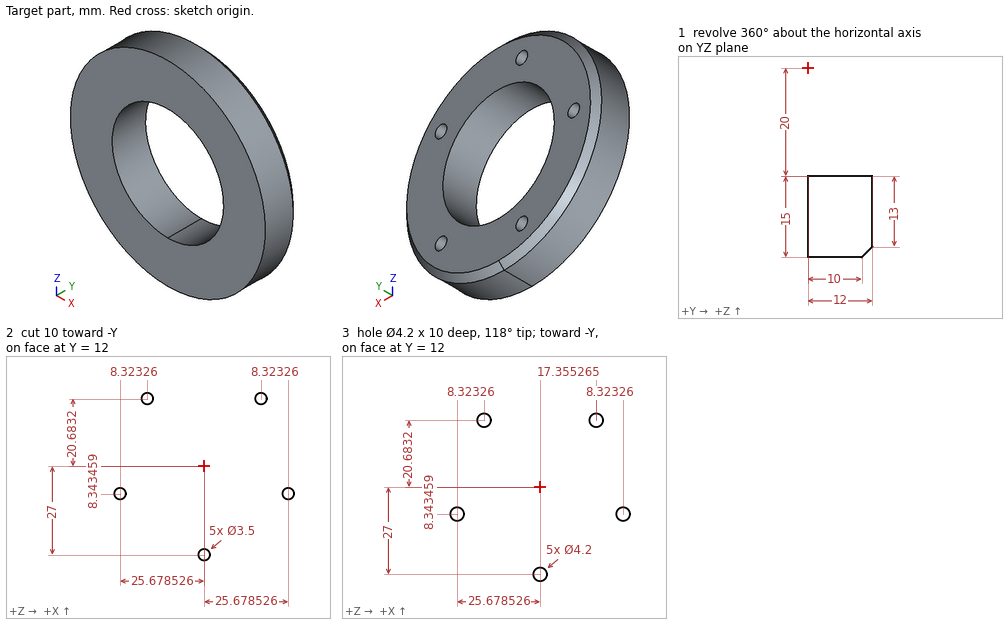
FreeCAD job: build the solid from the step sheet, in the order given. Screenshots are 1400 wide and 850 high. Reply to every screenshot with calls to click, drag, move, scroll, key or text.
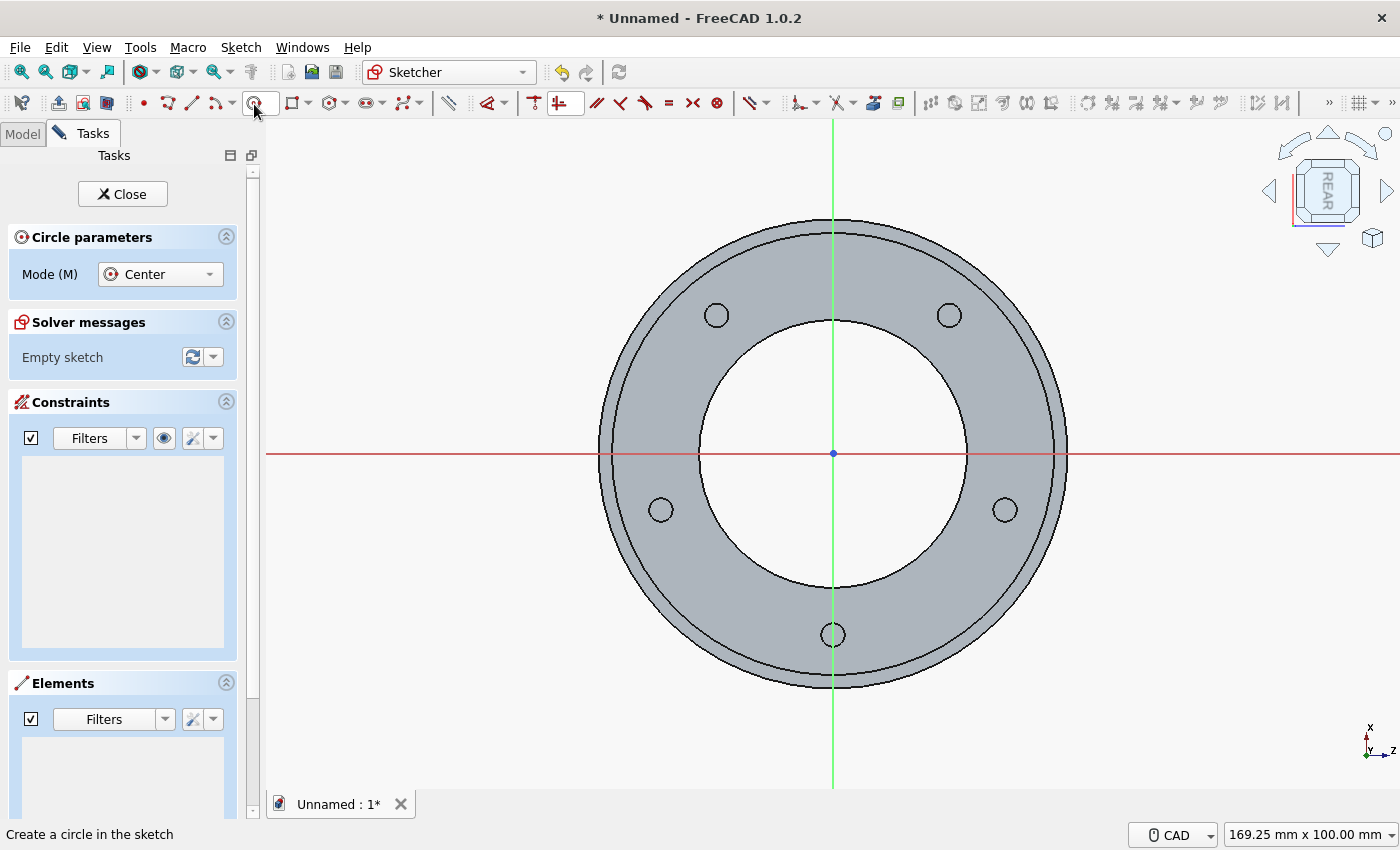
scroll(833, 635, up, 3)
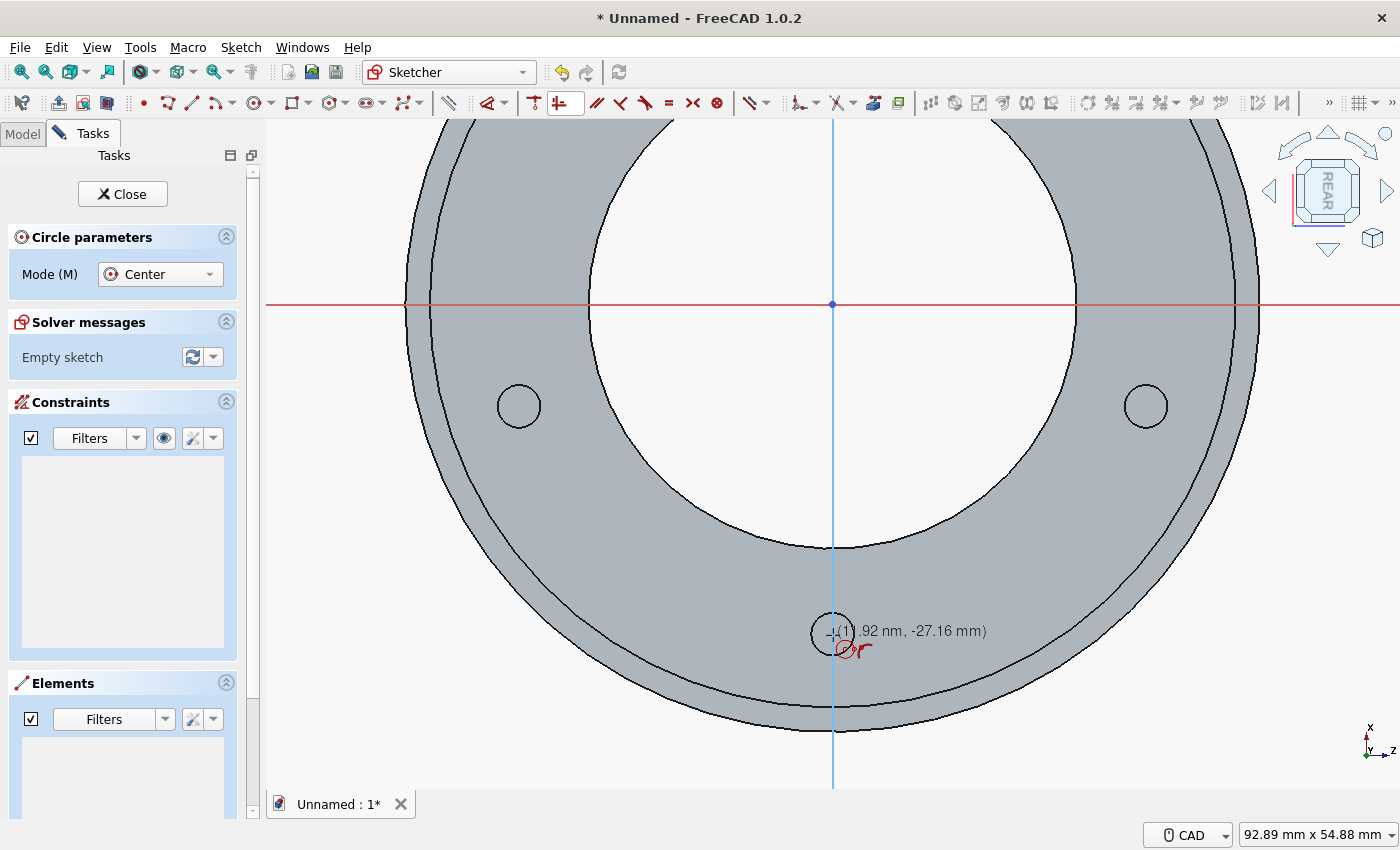
click(833, 634)
click(851, 616)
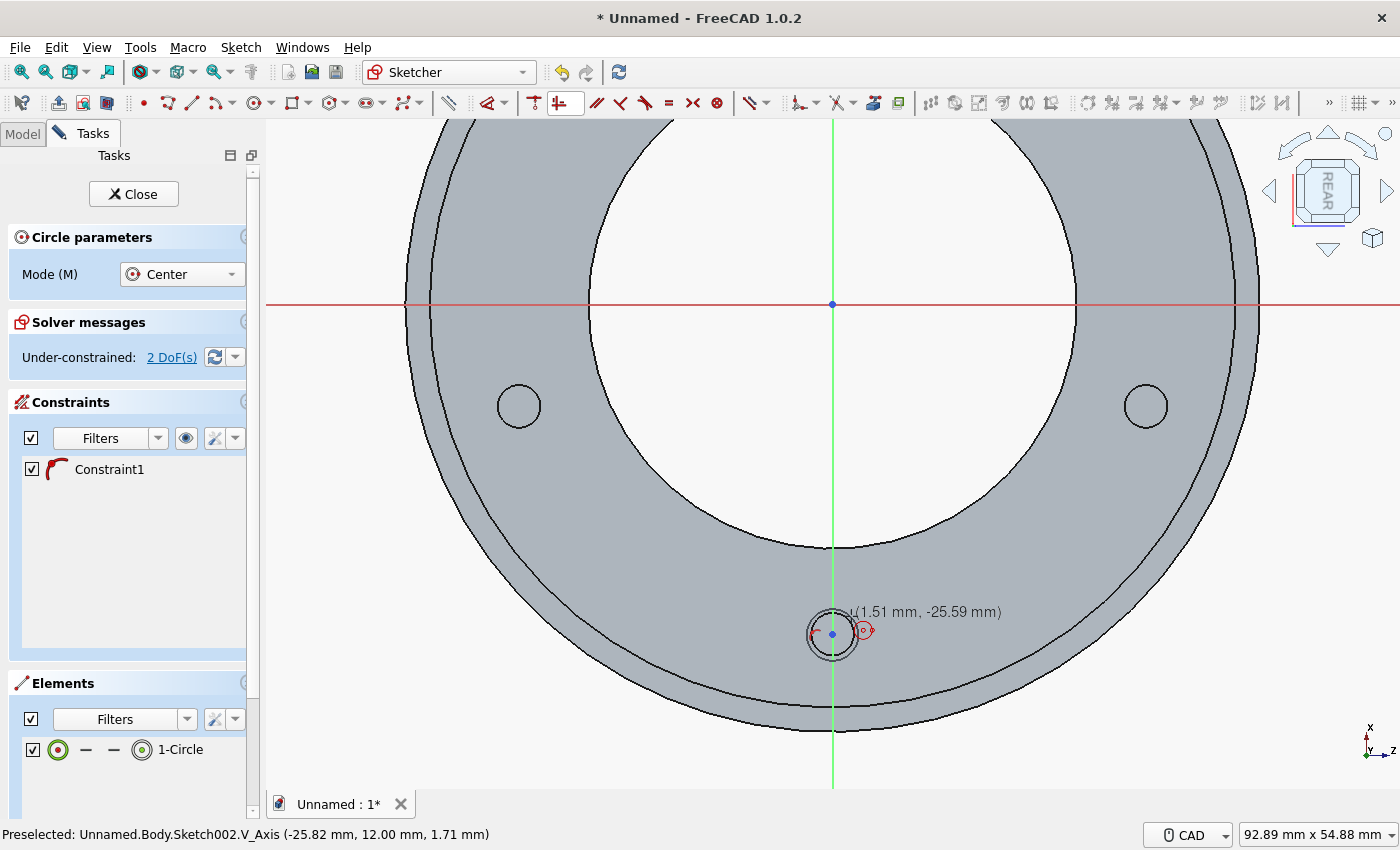
click(519, 406)
click(537, 388)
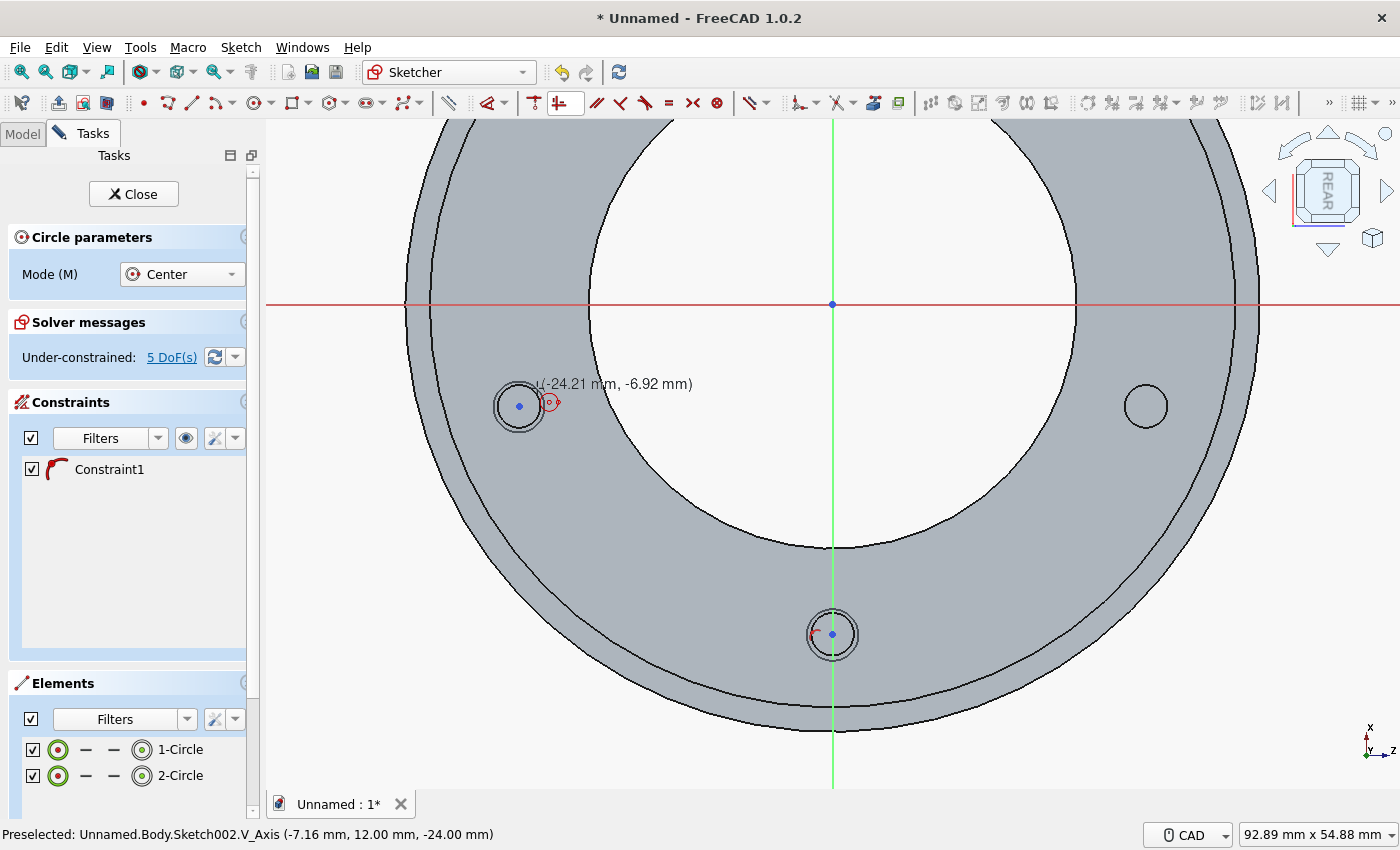
scroll(626, 679, down, 2)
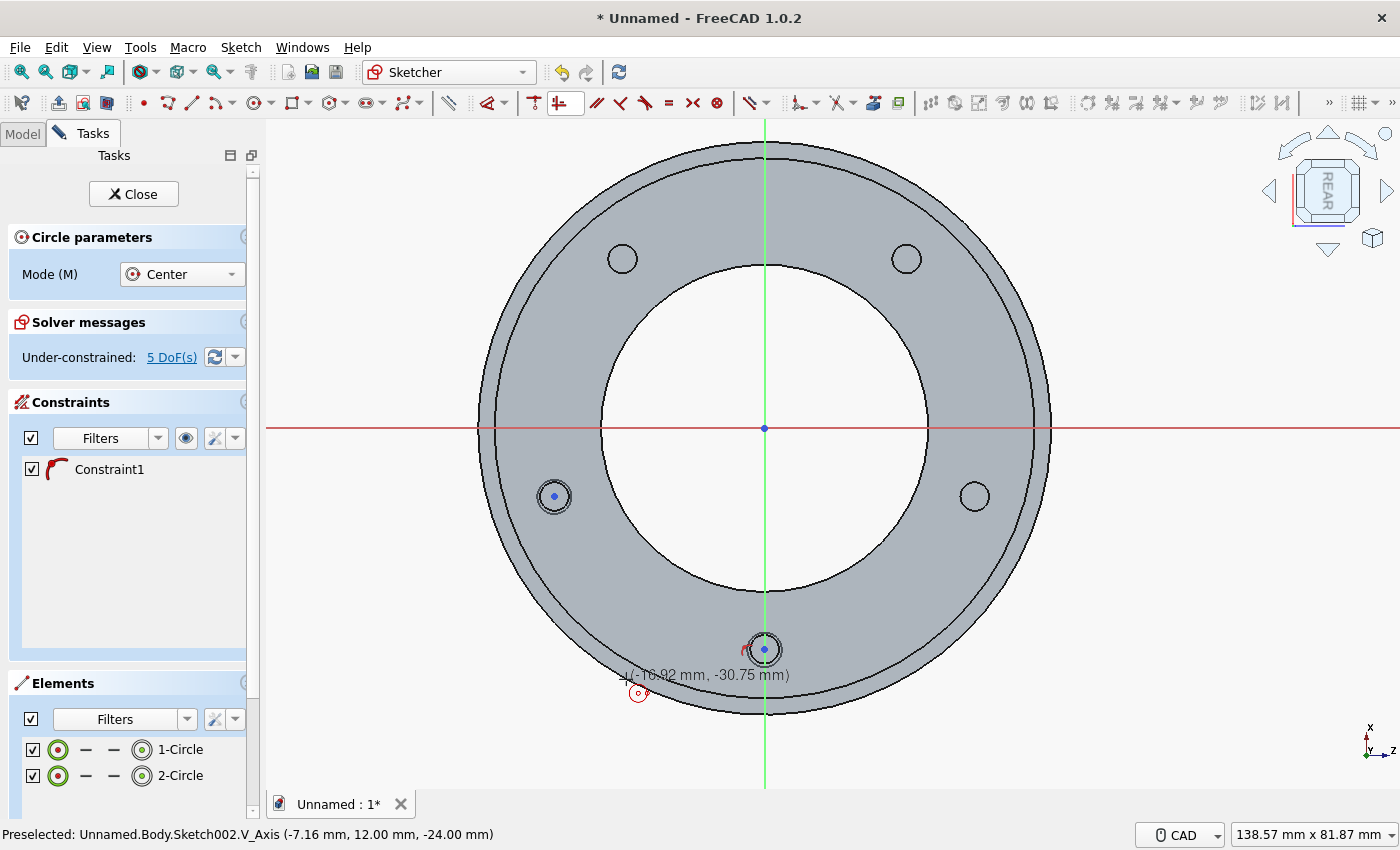
scroll(623, 259, up, 2)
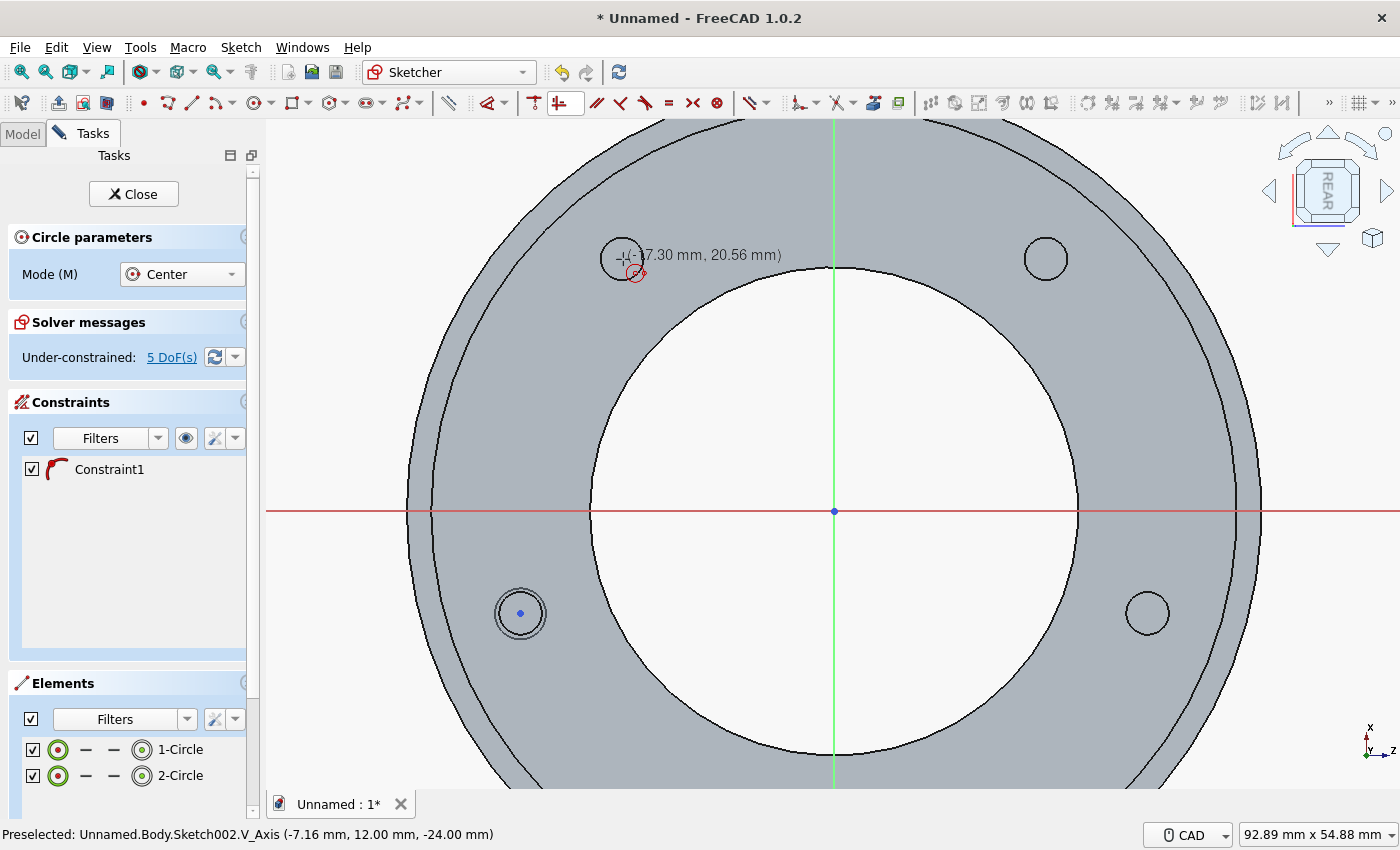
click(622, 259)
click(640, 241)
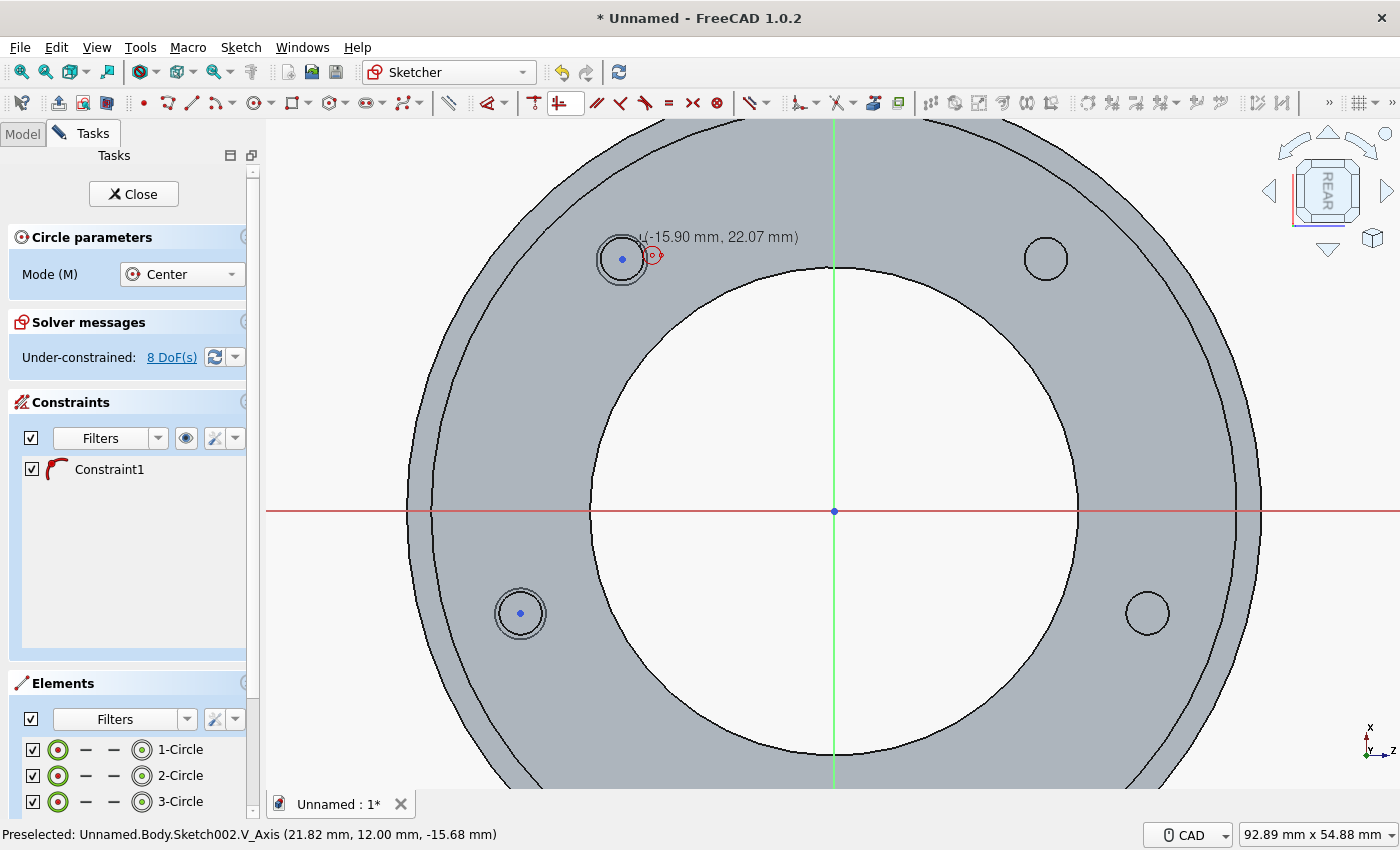
click(1046, 259)
click(1064, 241)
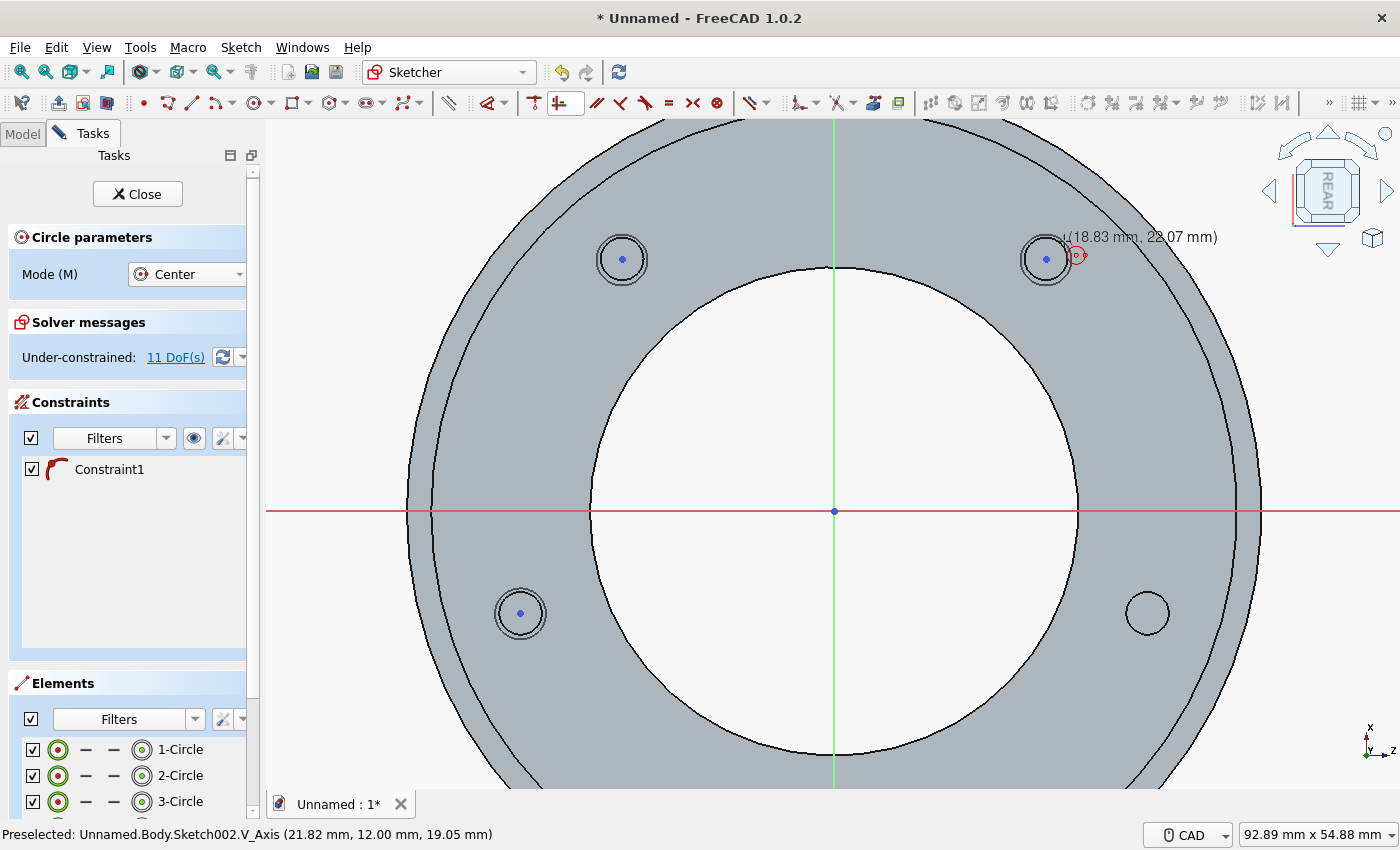
click(1148, 613)
click(1166, 595)
key(Escape)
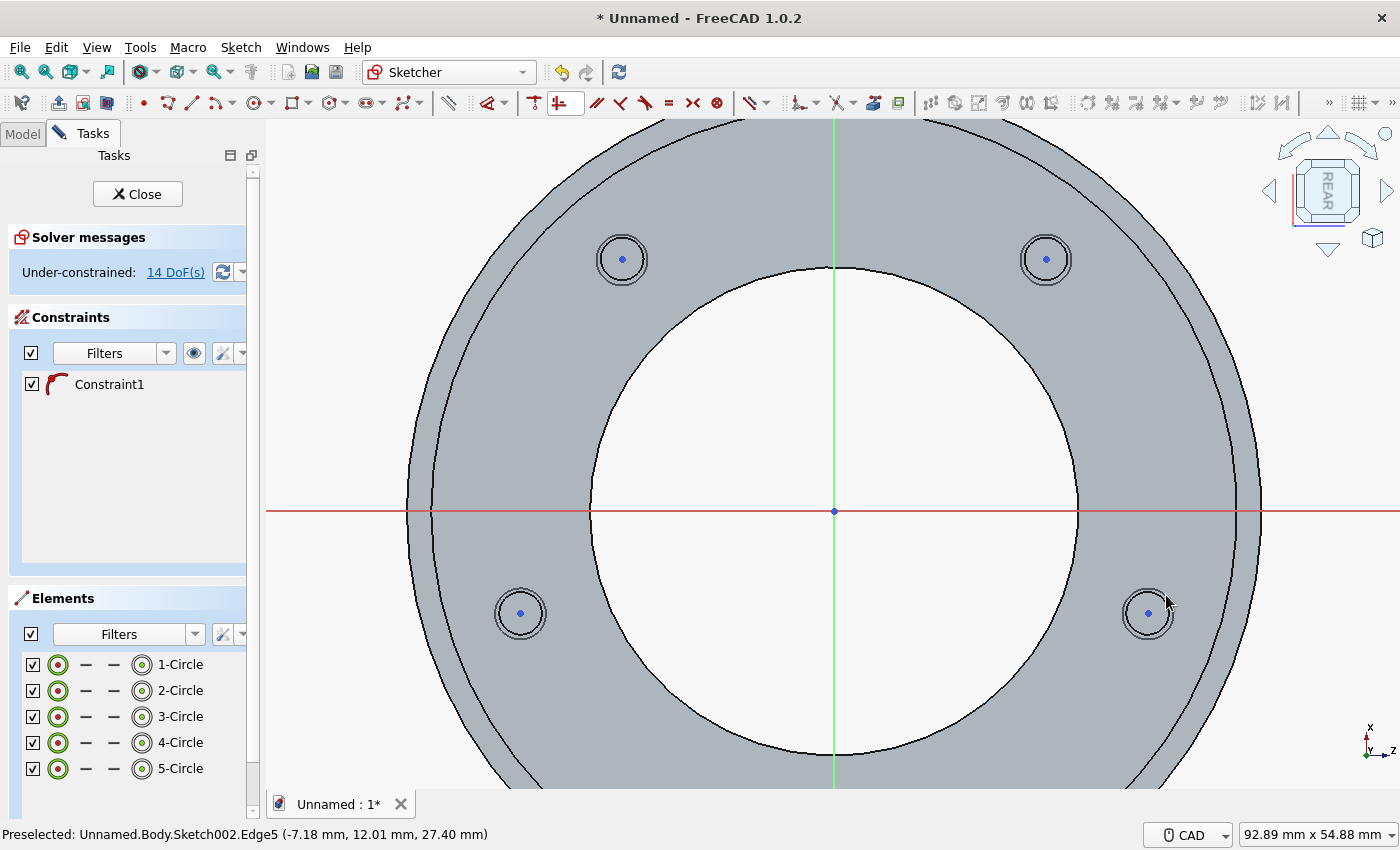
scroll(623, 259, down, 2)